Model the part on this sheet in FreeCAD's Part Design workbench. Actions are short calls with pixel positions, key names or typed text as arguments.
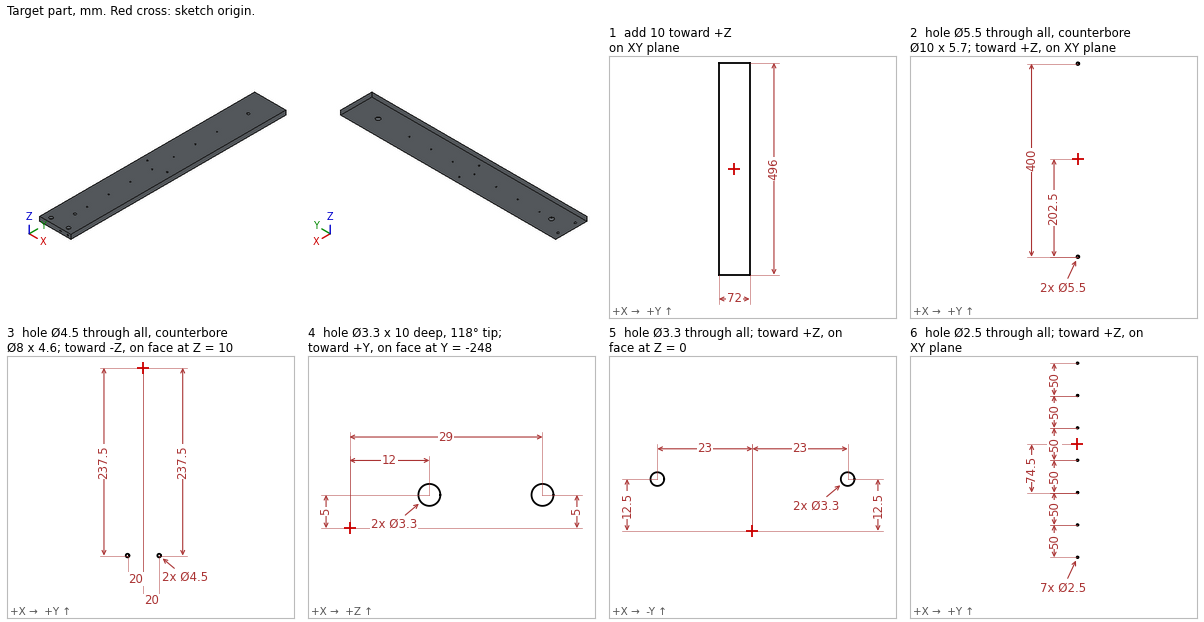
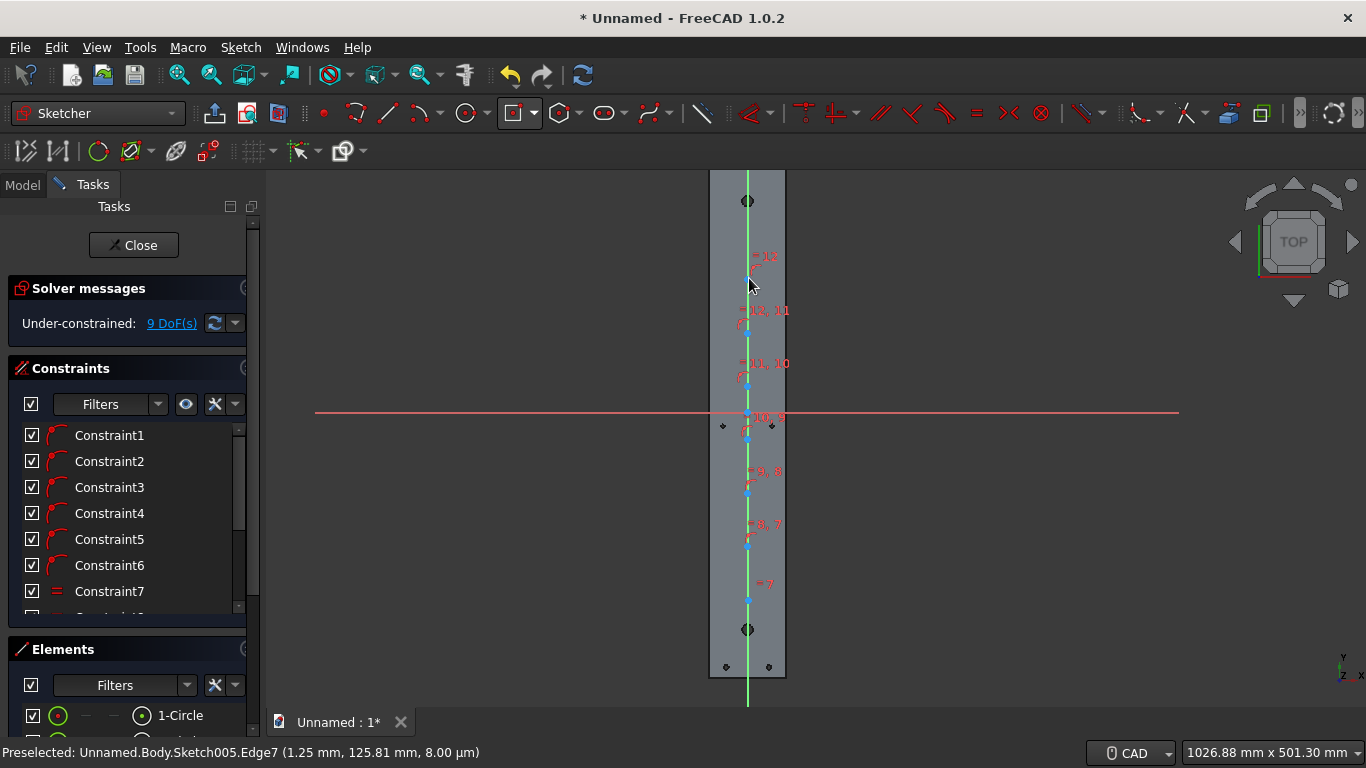
click(748, 601)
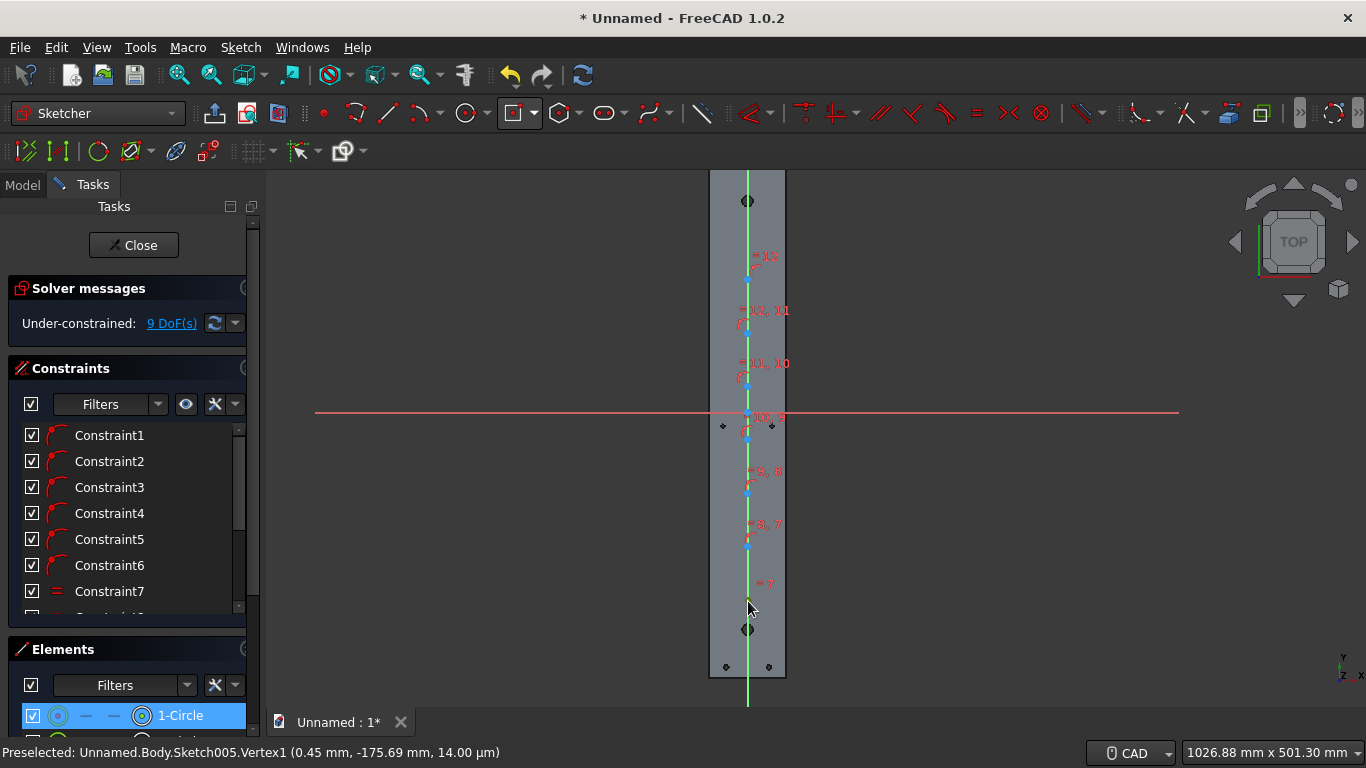
click(748, 645)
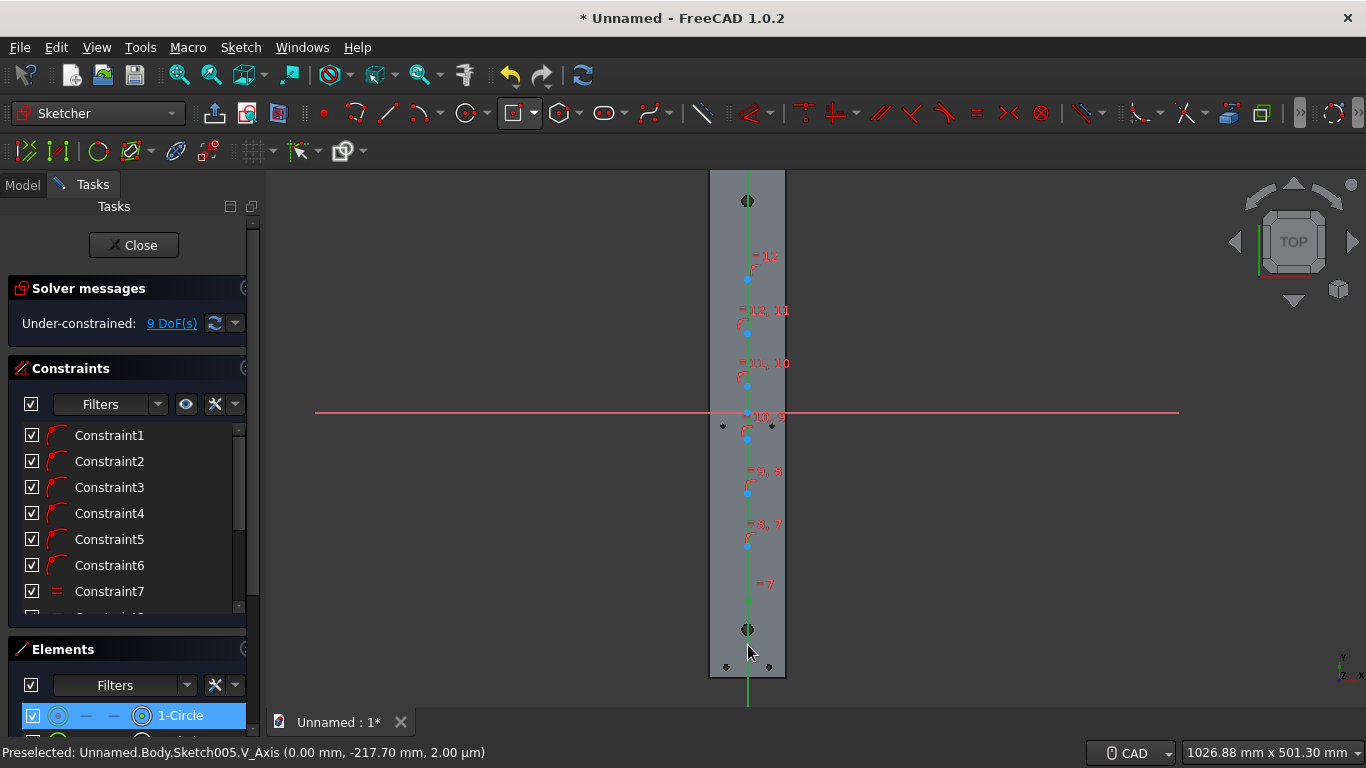
click(804, 114)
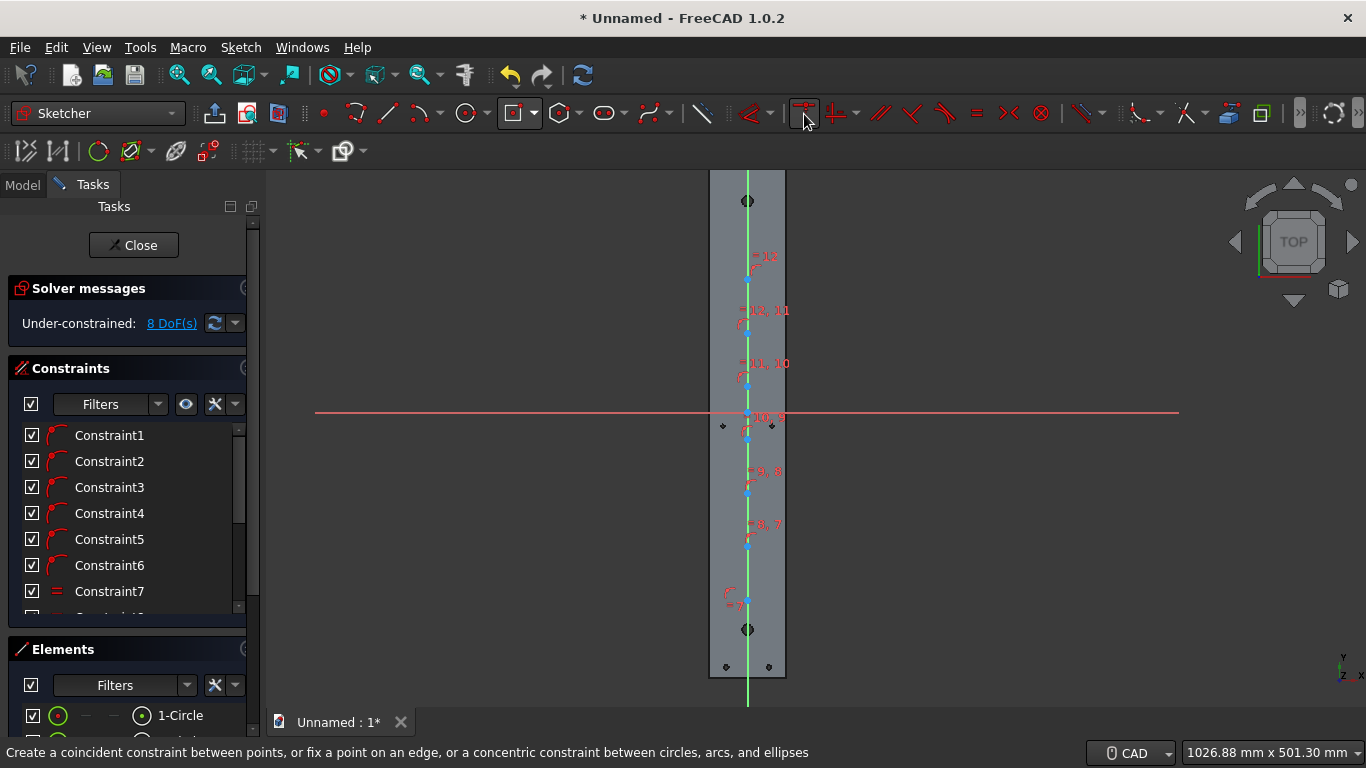
key(d)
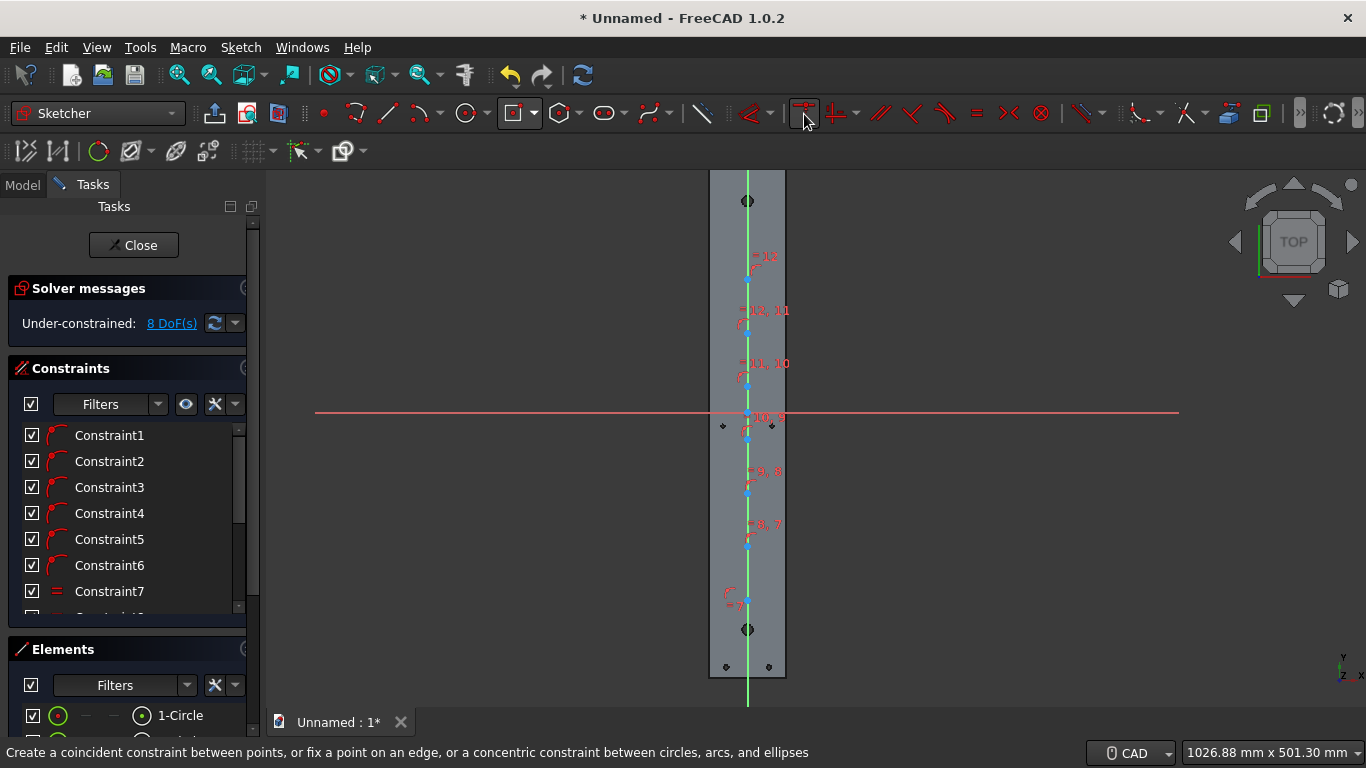
scroll(748, 599, up, 14)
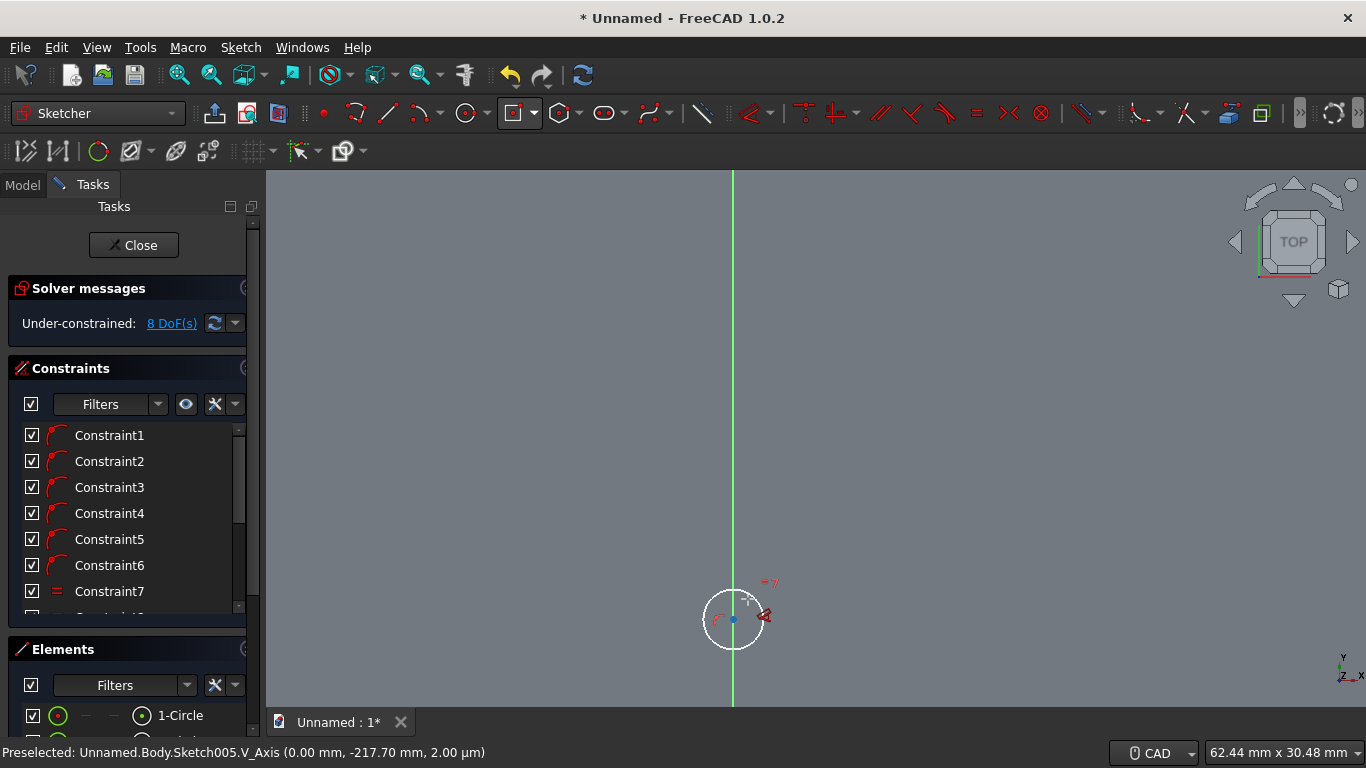
click(734, 590)
click(764, 566)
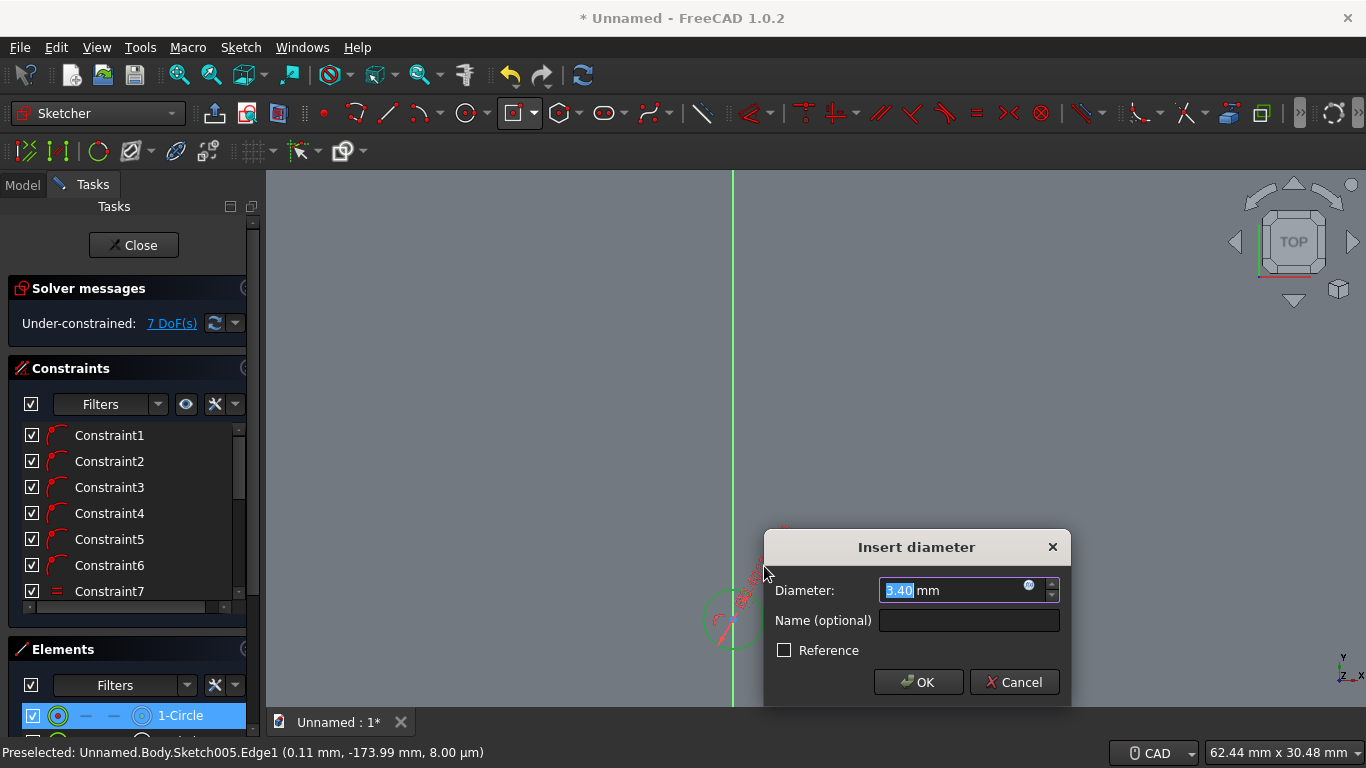
text(2.5)
key(Return)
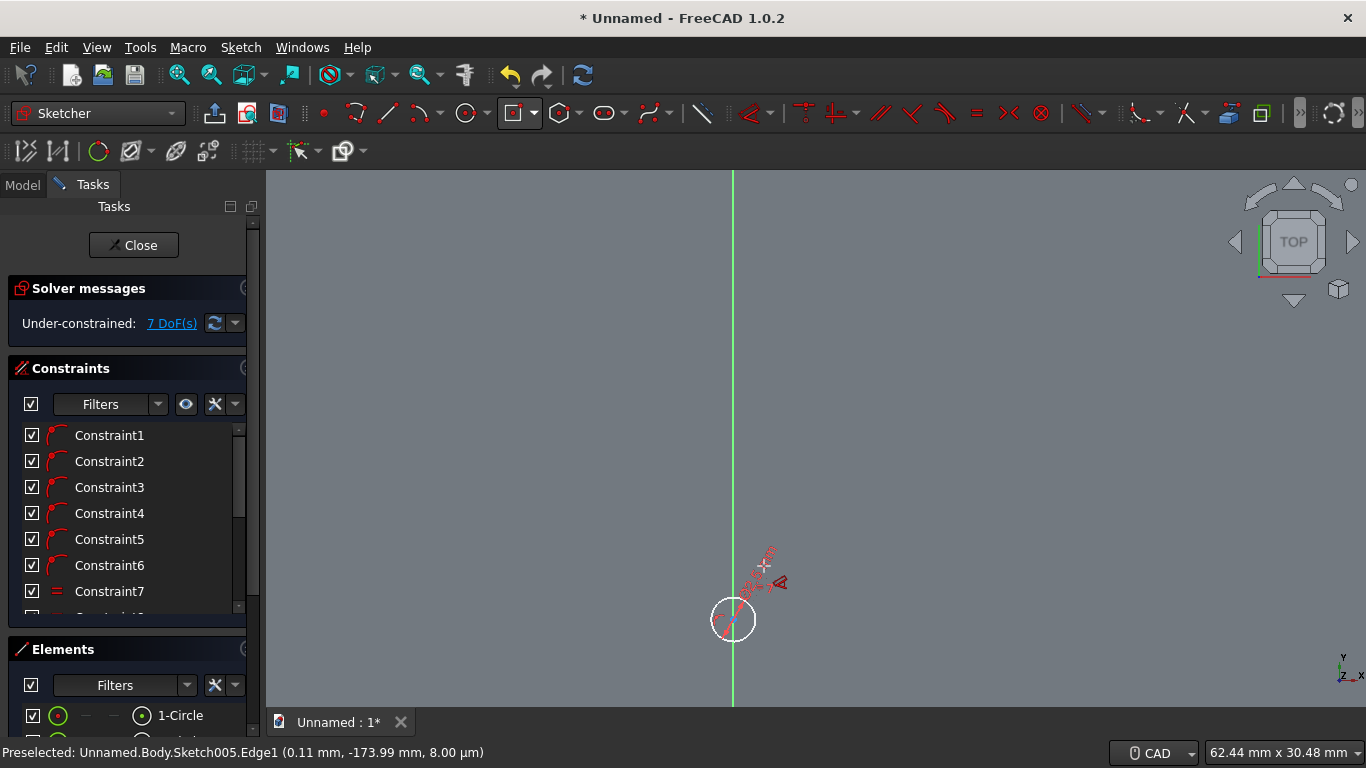
scroll(748, 599, down, 14)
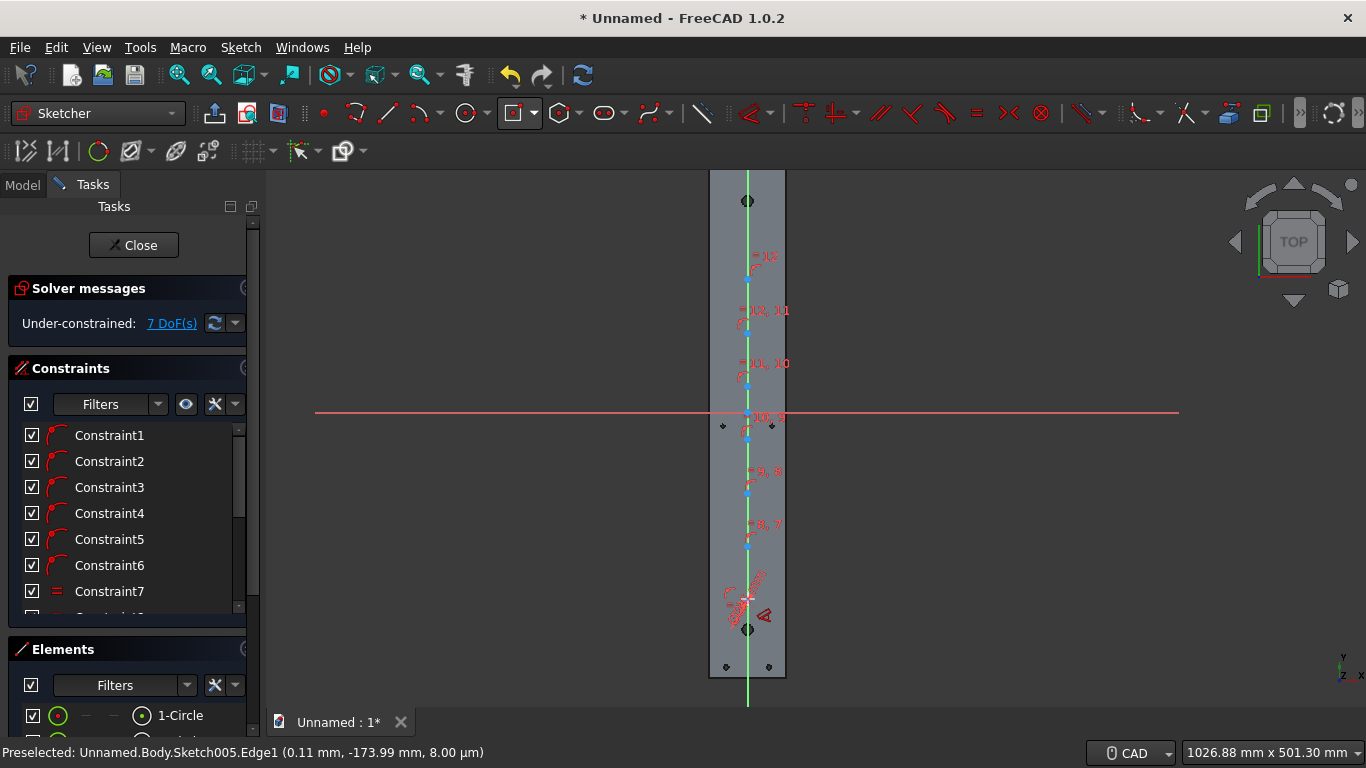
click(748, 601)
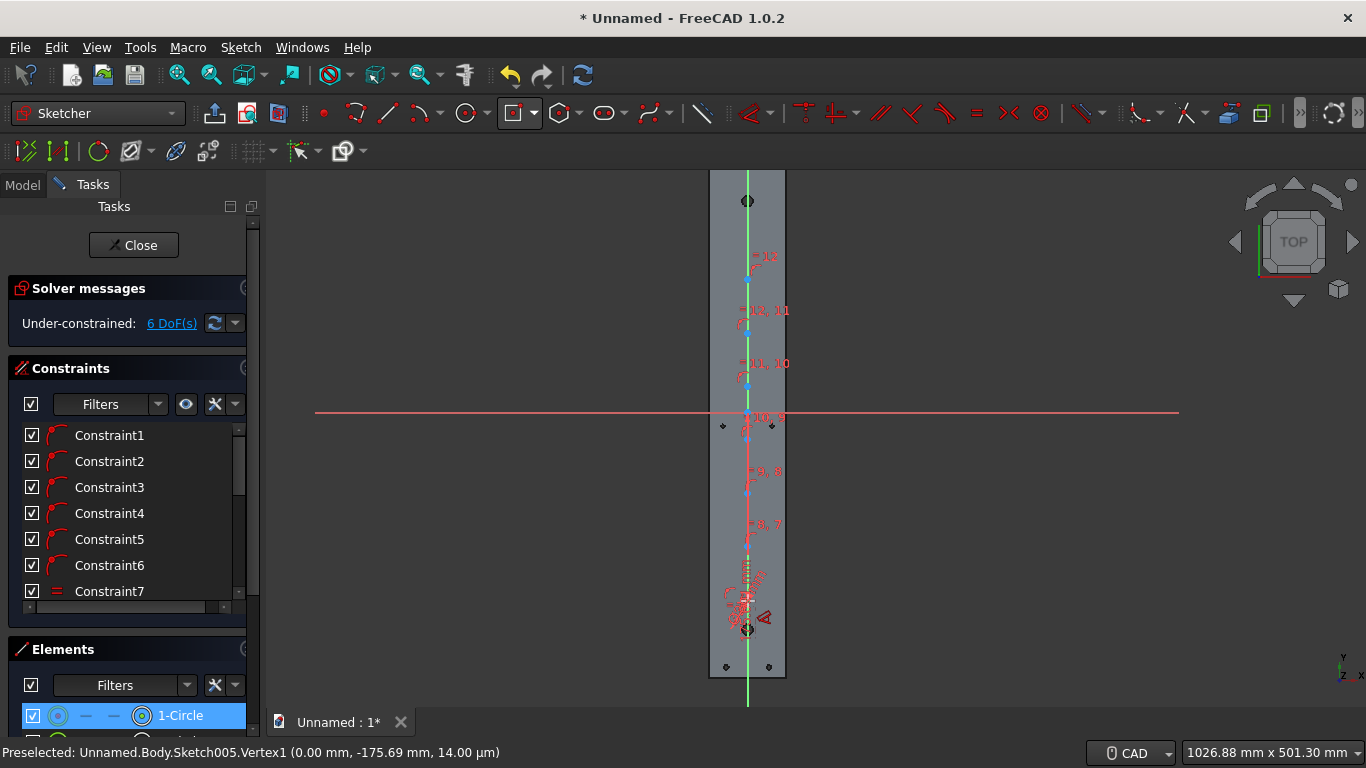
click(748, 547)
click(782, 574)